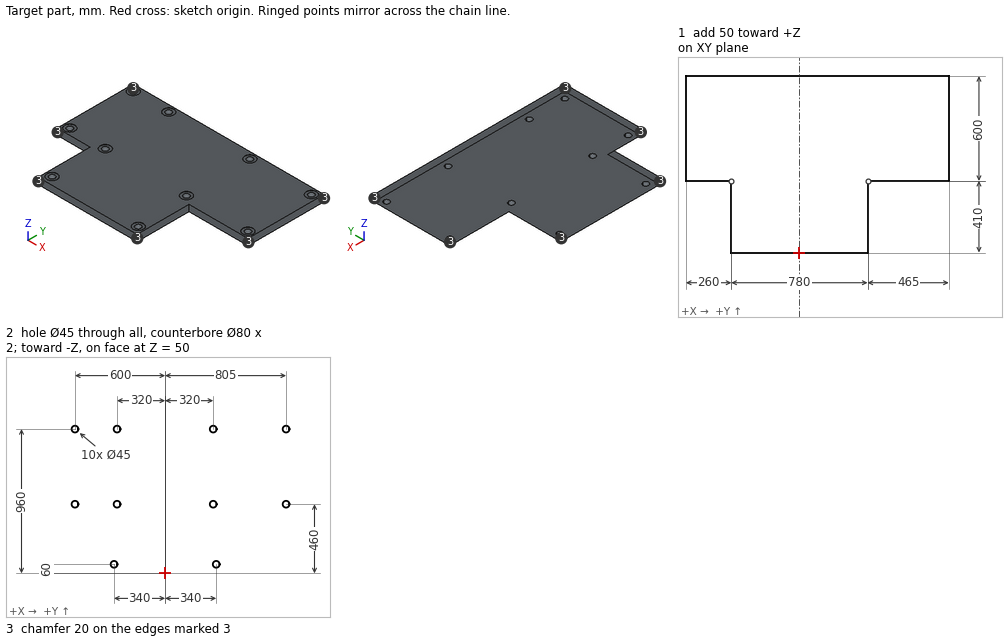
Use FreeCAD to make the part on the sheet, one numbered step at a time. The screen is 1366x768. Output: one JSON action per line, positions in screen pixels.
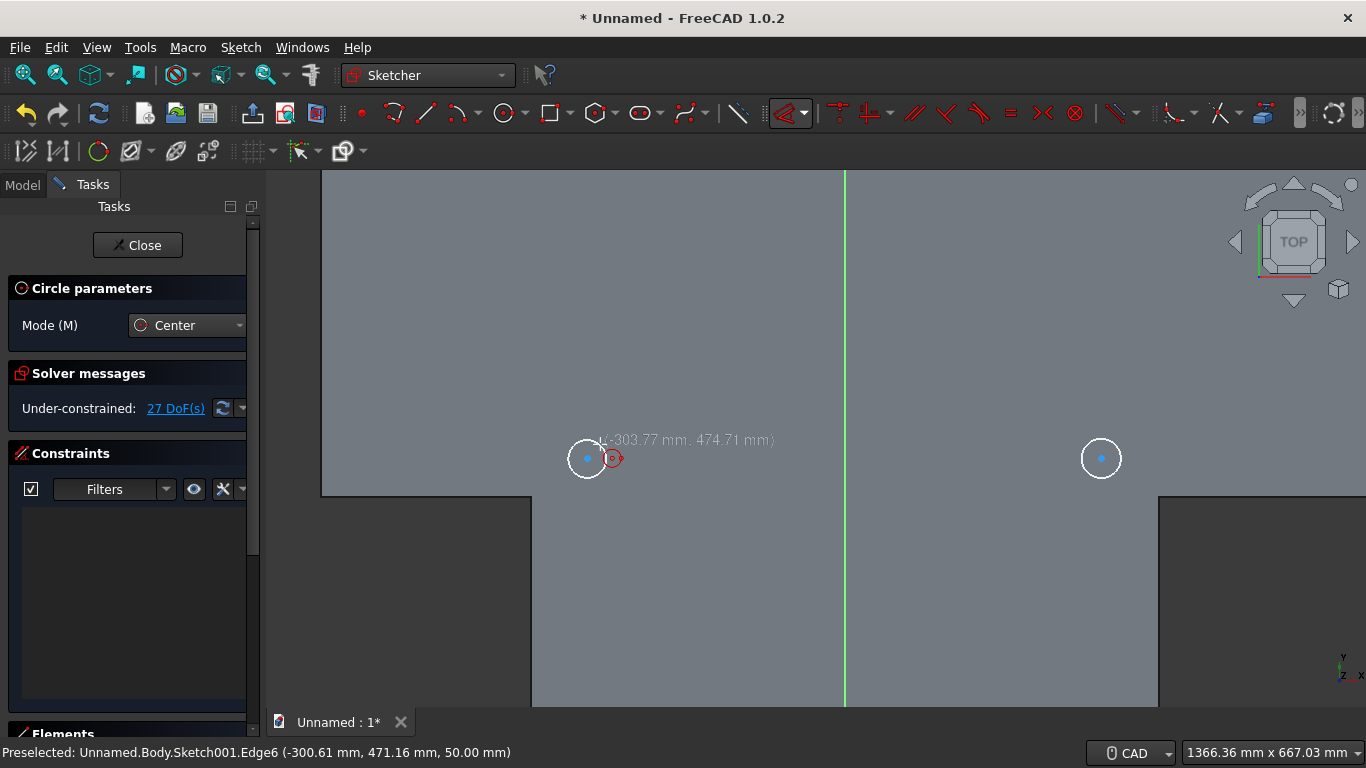
{"action": "scroll", "coordinate": [362, 457], "scroll_direction": "up", "scroll_amount": 2}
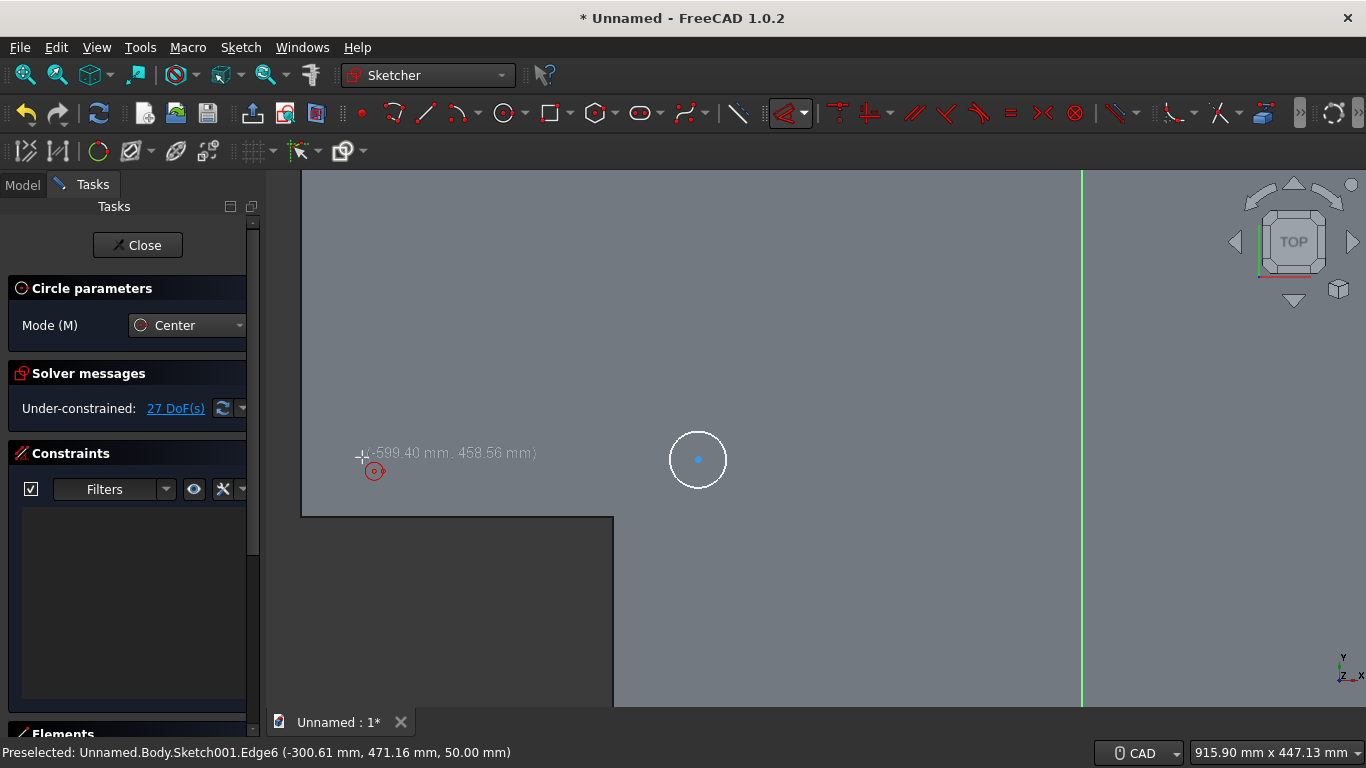
{"action": "scroll", "coordinate": [550, 447], "scroll_direction": "down", "scroll_amount": 6}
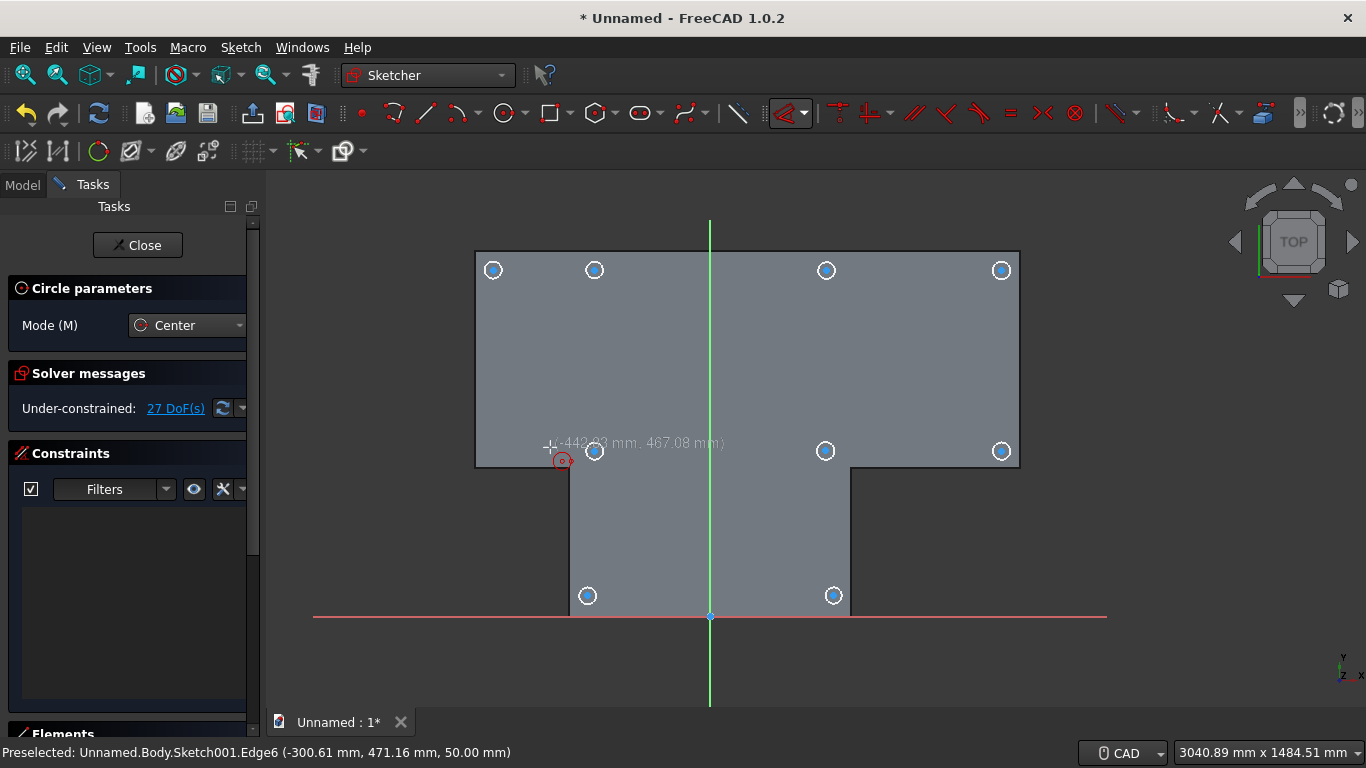
{"action": "left_click", "coordinate": [493, 450]}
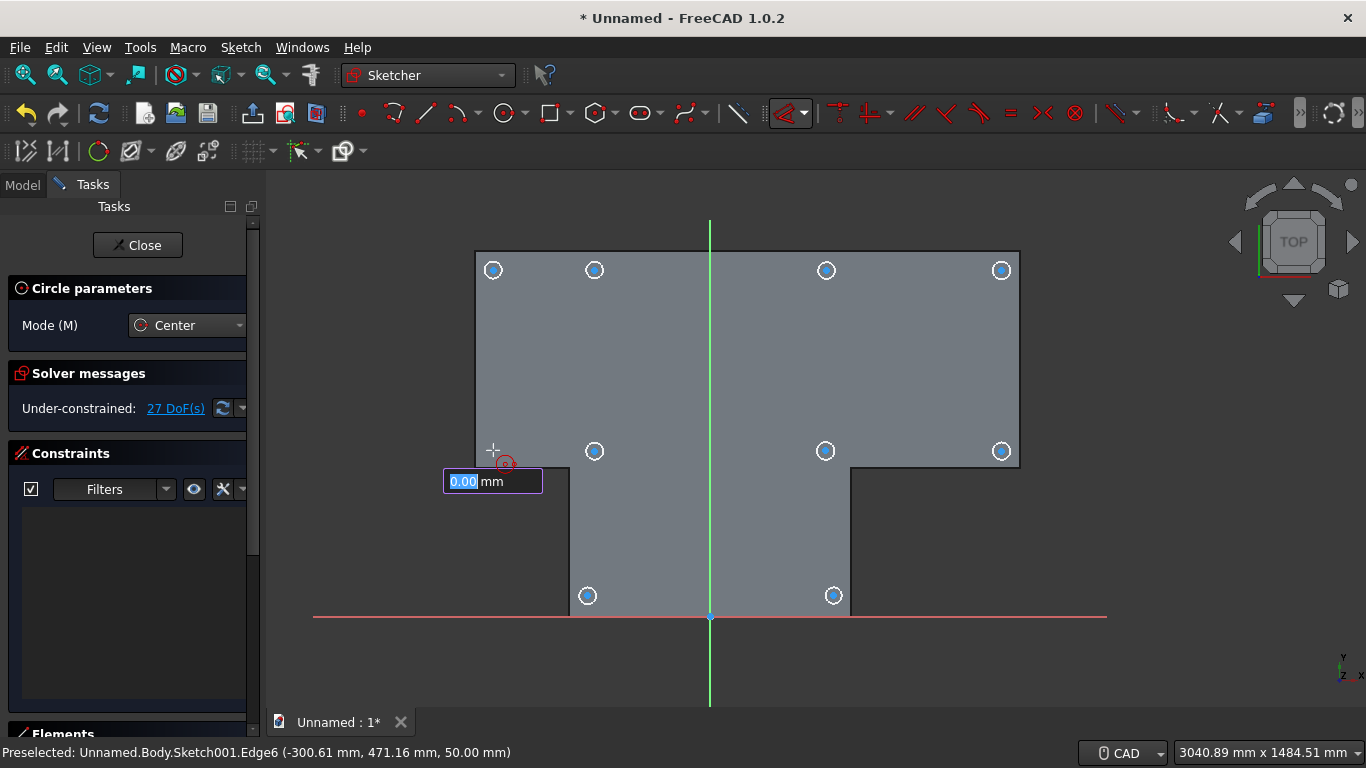
{"action": "scroll", "coordinate": [499, 444], "scroll_direction": "up", "scroll_amount": 4}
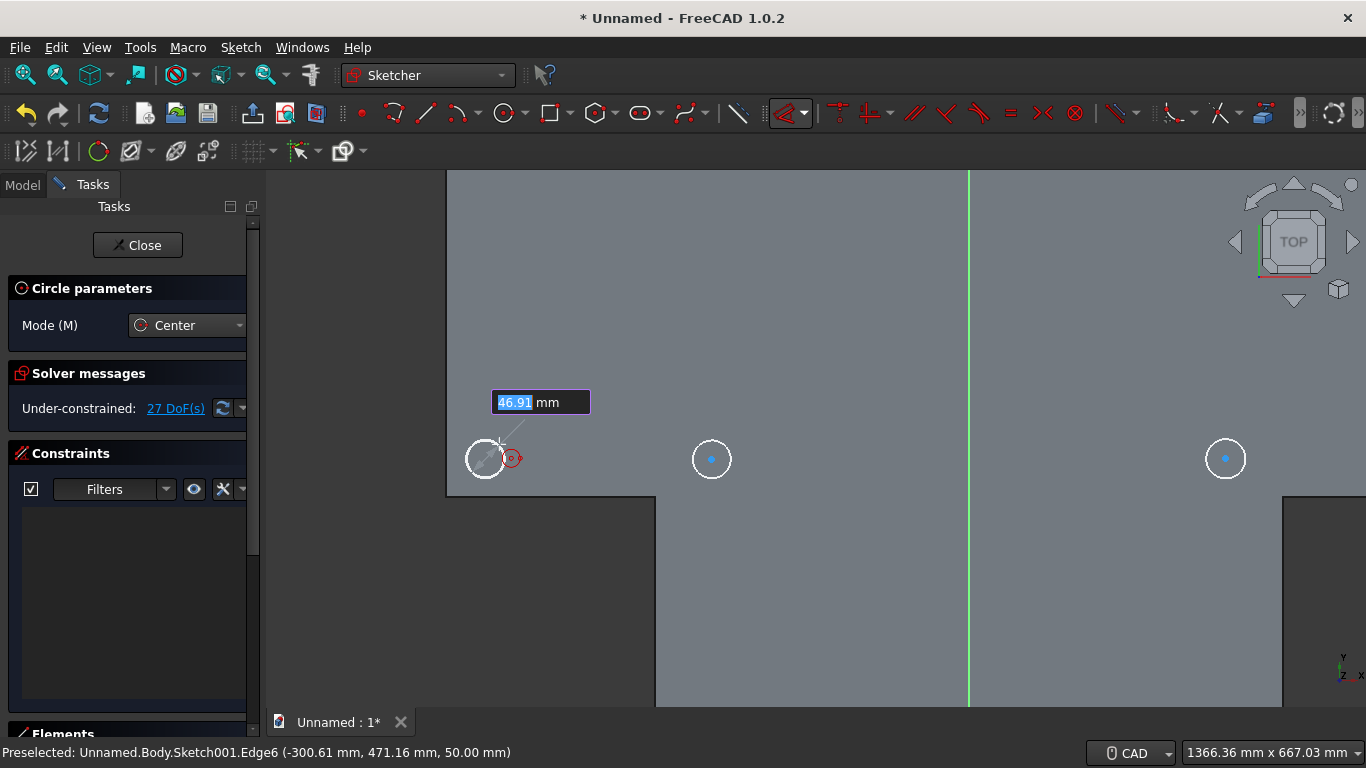
{"action": "left_click", "coordinate": [499, 444]}
{"action": "key", "text": "Escape"}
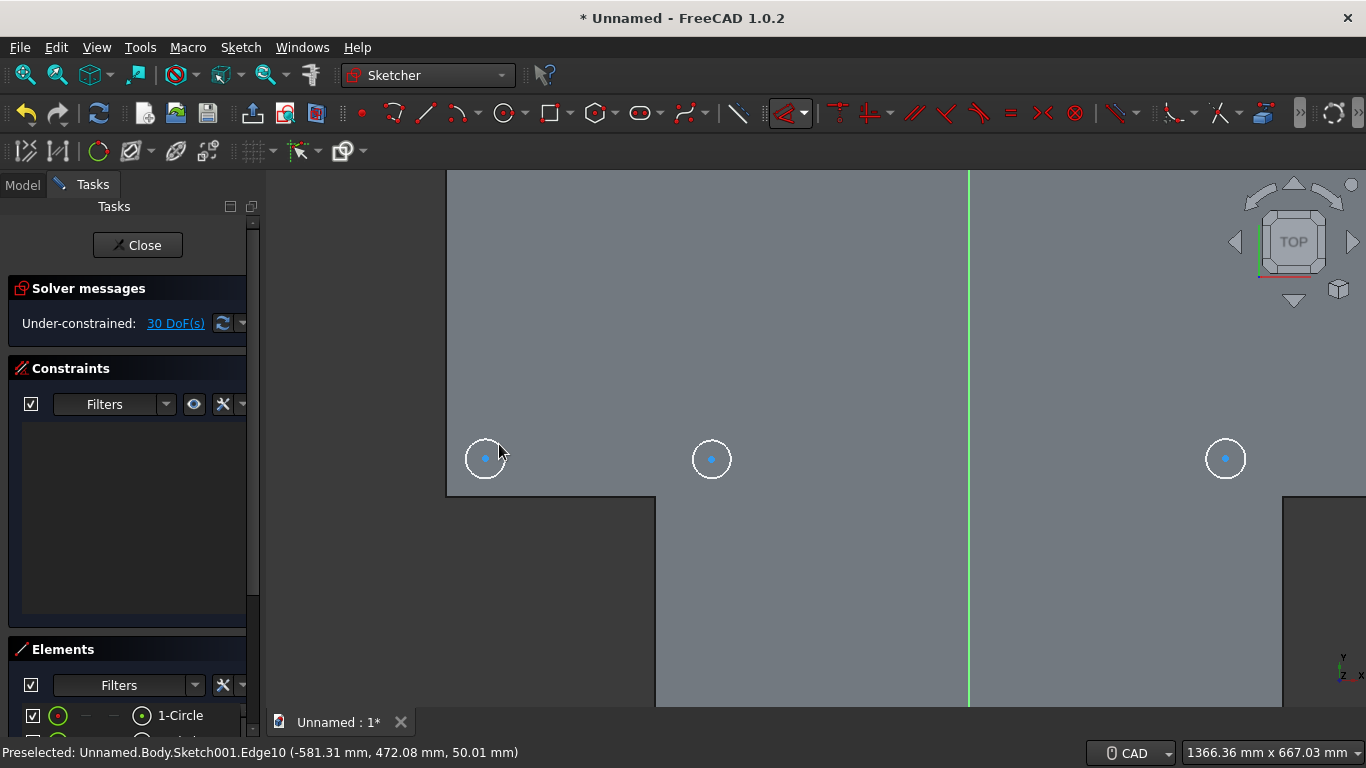
{"action": "scroll", "coordinate": [499, 444], "scroll_direction": "down", "scroll_amount": 4}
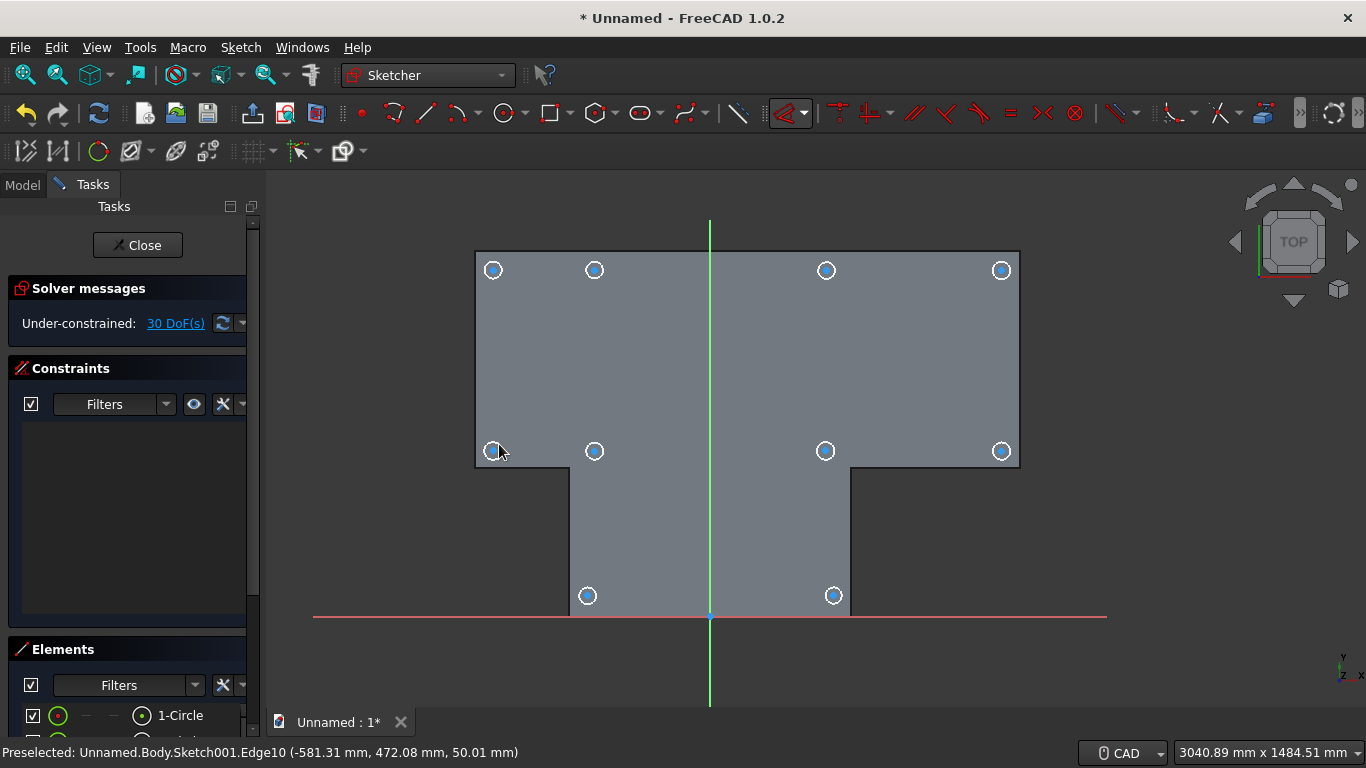
{"action": "scroll", "coordinate": [499, 264], "scroll_direction": "up", "scroll_amount": 3}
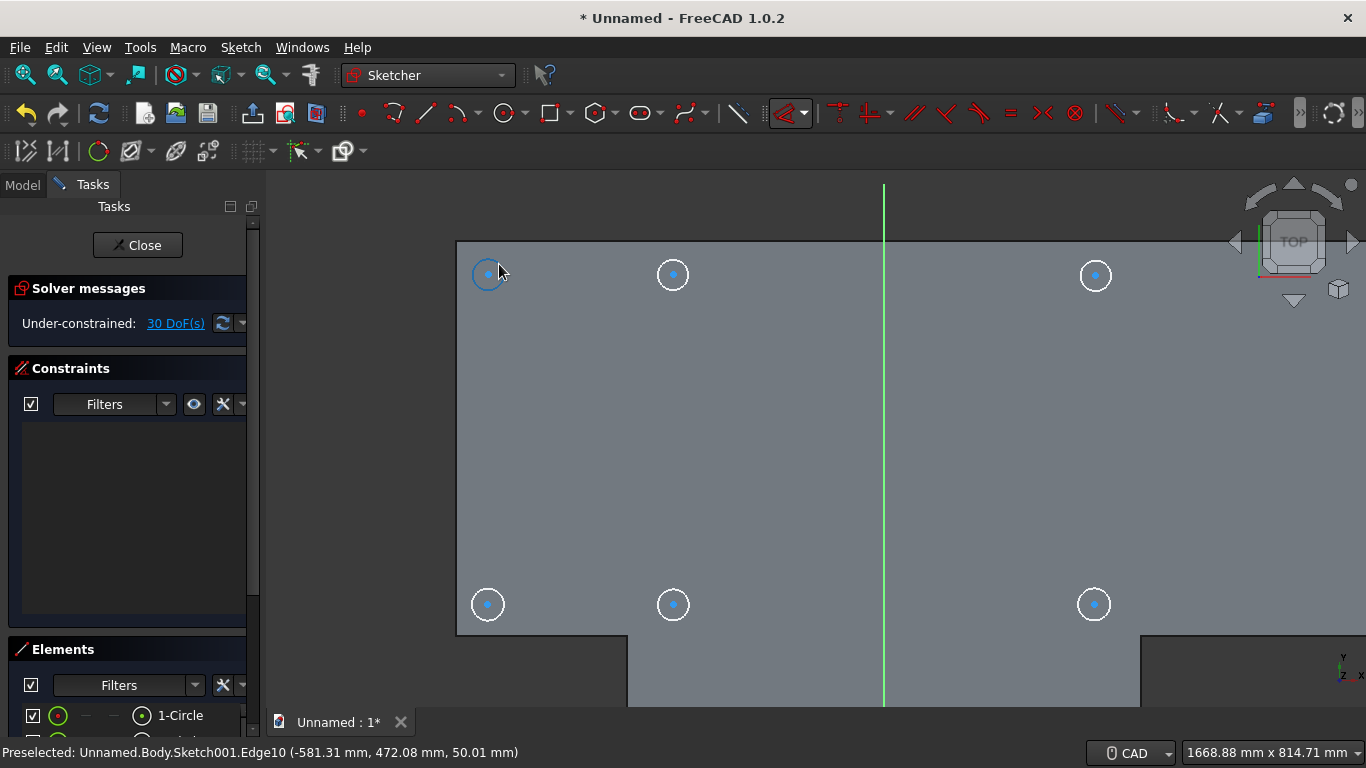
{"action": "left_click", "coordinate": [499, 264]}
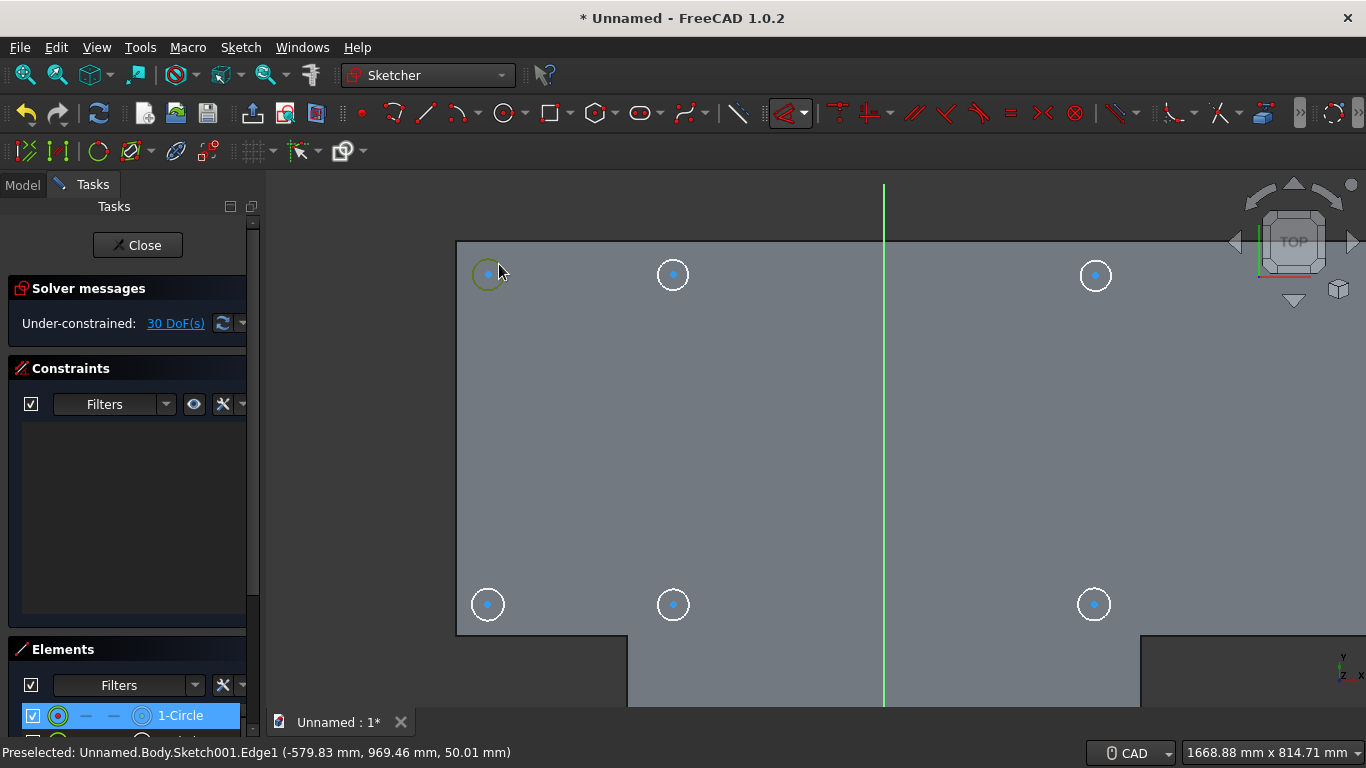
{"action": "left_click", "coordinate": [1107, 265]}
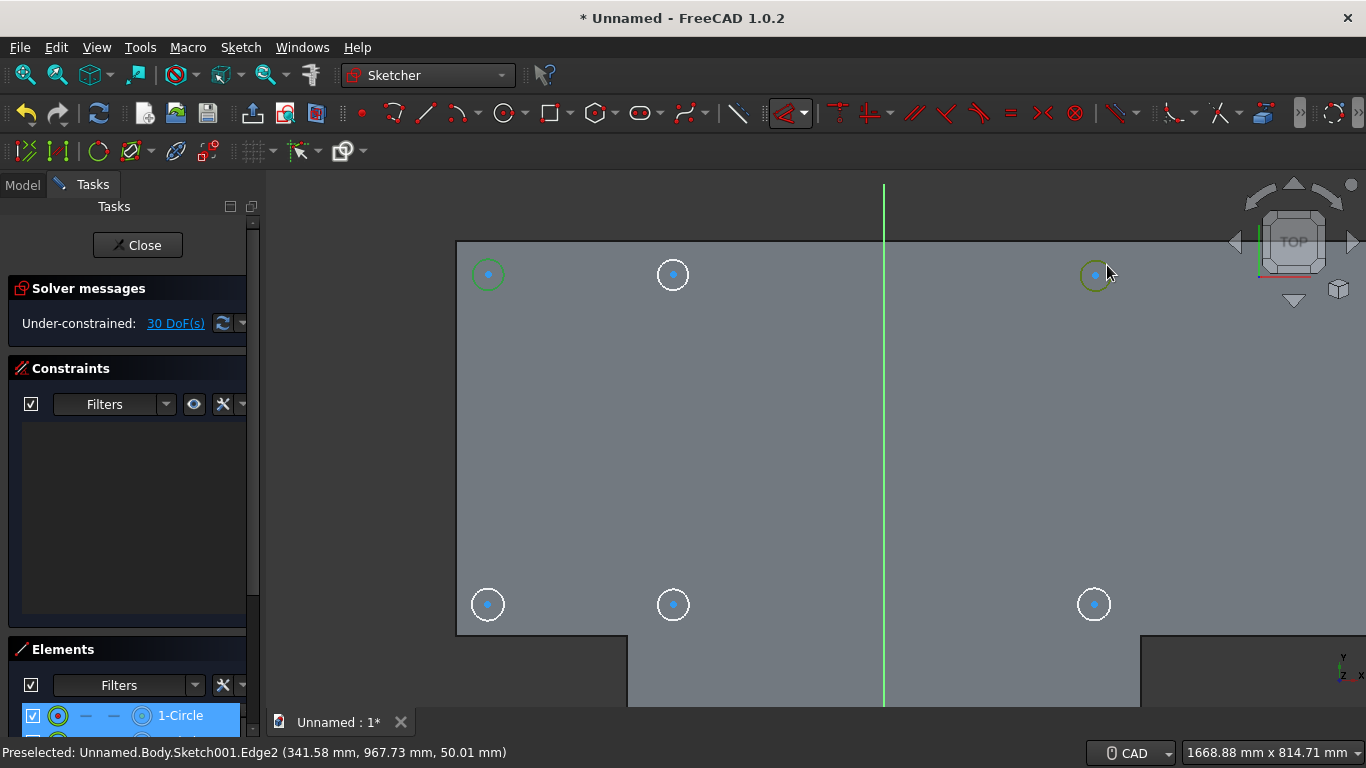
{"action": "scroll", "coordinate": [499, 263], "scroll_direction": "down", "scroll_amount": 3}